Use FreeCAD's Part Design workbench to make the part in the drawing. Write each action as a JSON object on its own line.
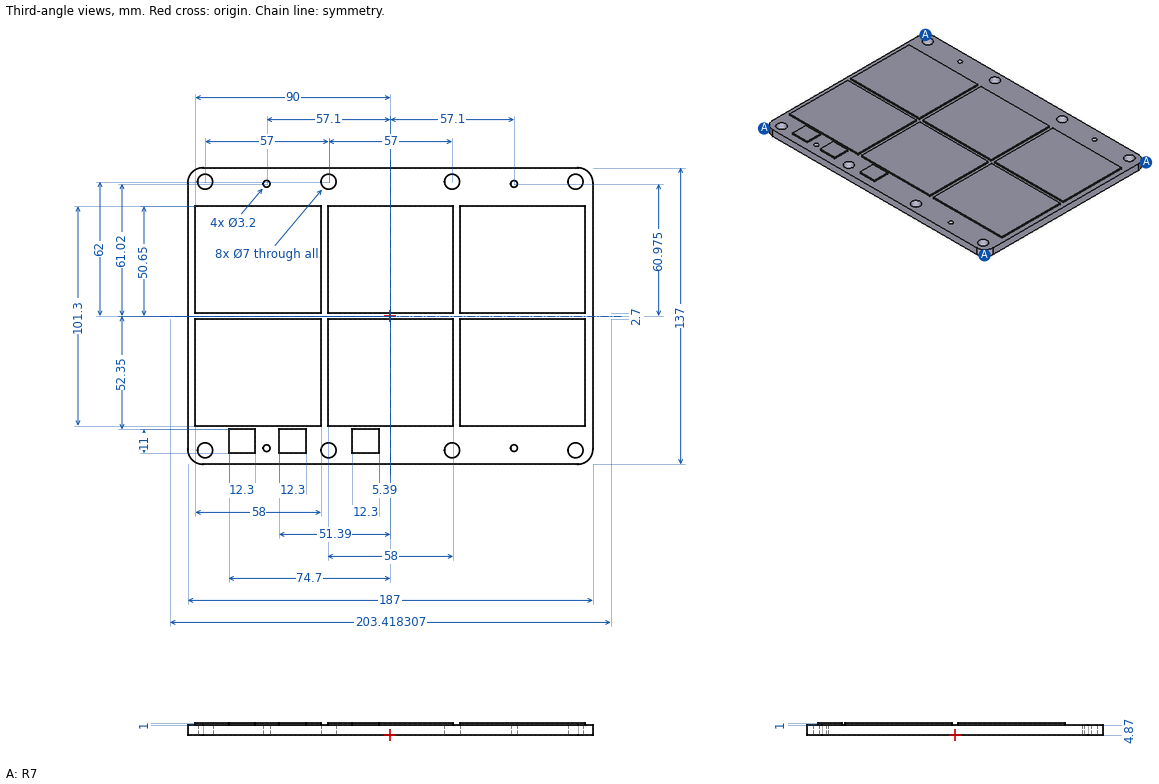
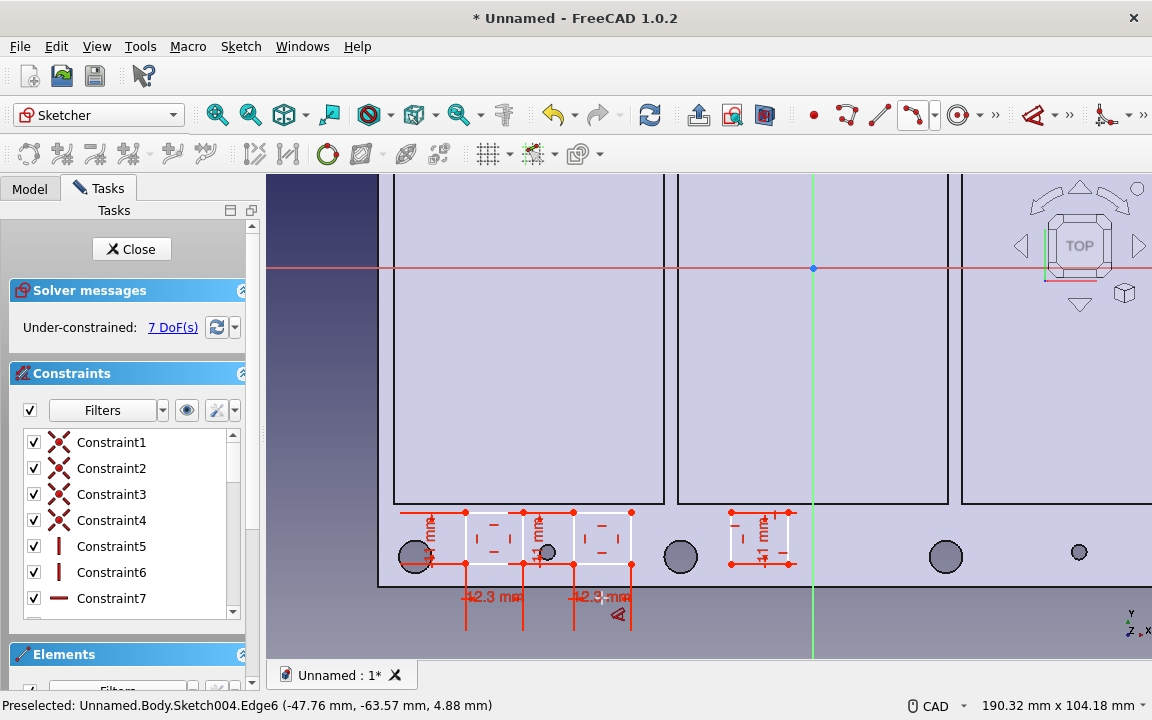
{"action": "left_click", "coordinate": [748, 564]}
{"action": "left_click", "coordinate": [760, 598]}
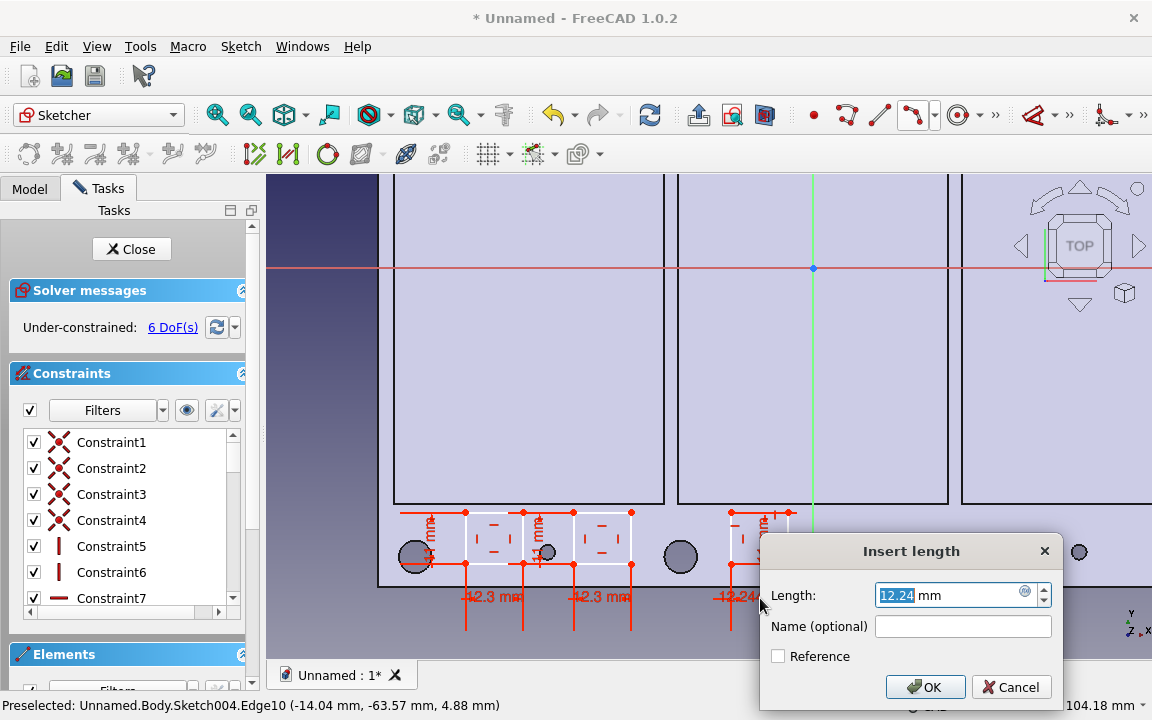
{"action": "type", "text": "12.3"}
{"action": "key", "text": "Return"}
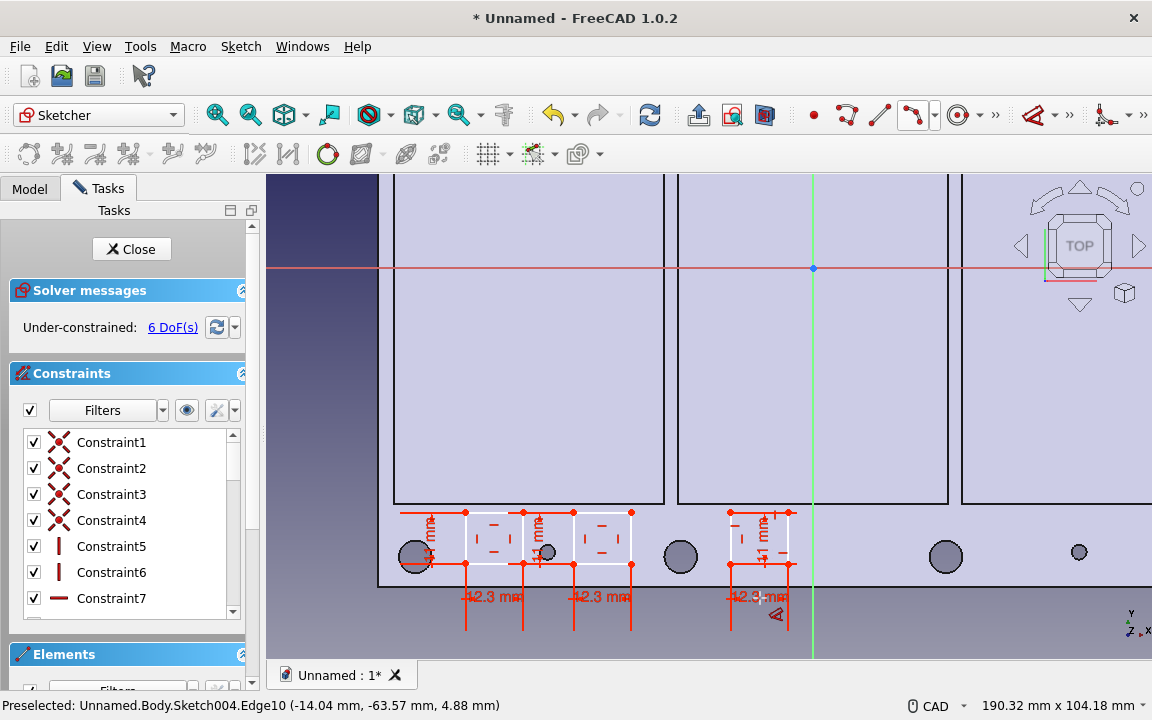
{"action": "left_click", "coordinate": [466, 513]}
{"action": "left_click", "coordinate": [640, 234]}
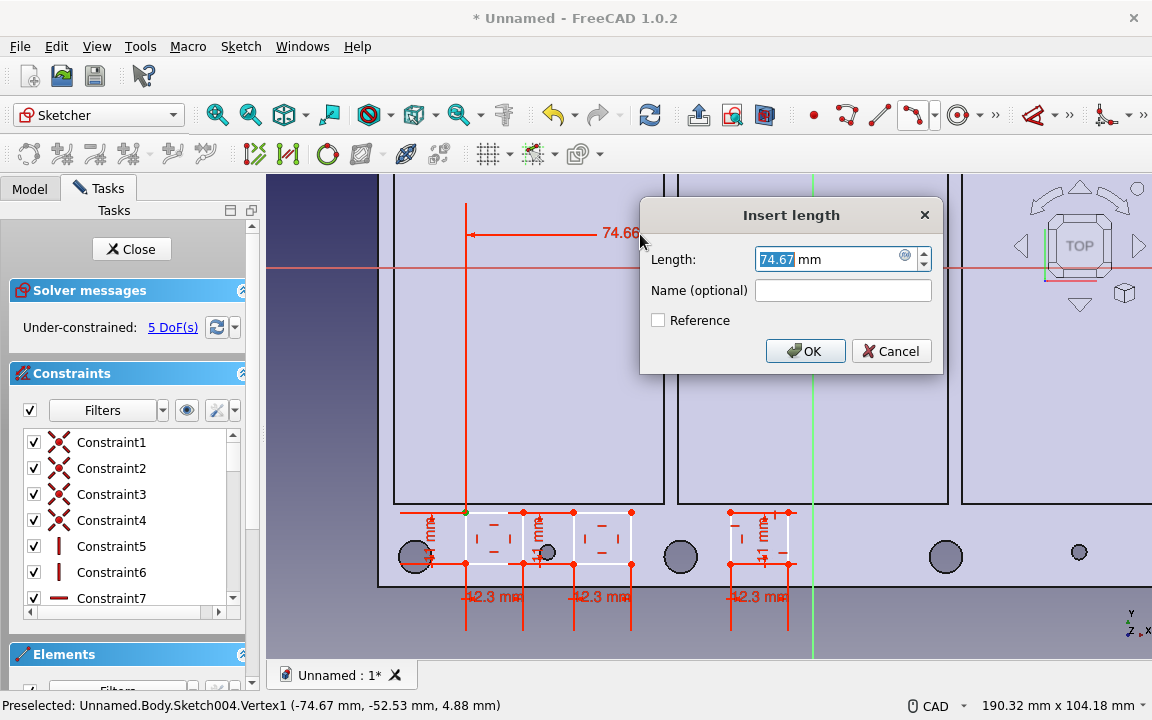
{"action": "type", "text": "74.7"}
{"action": "key", "text": "Return"}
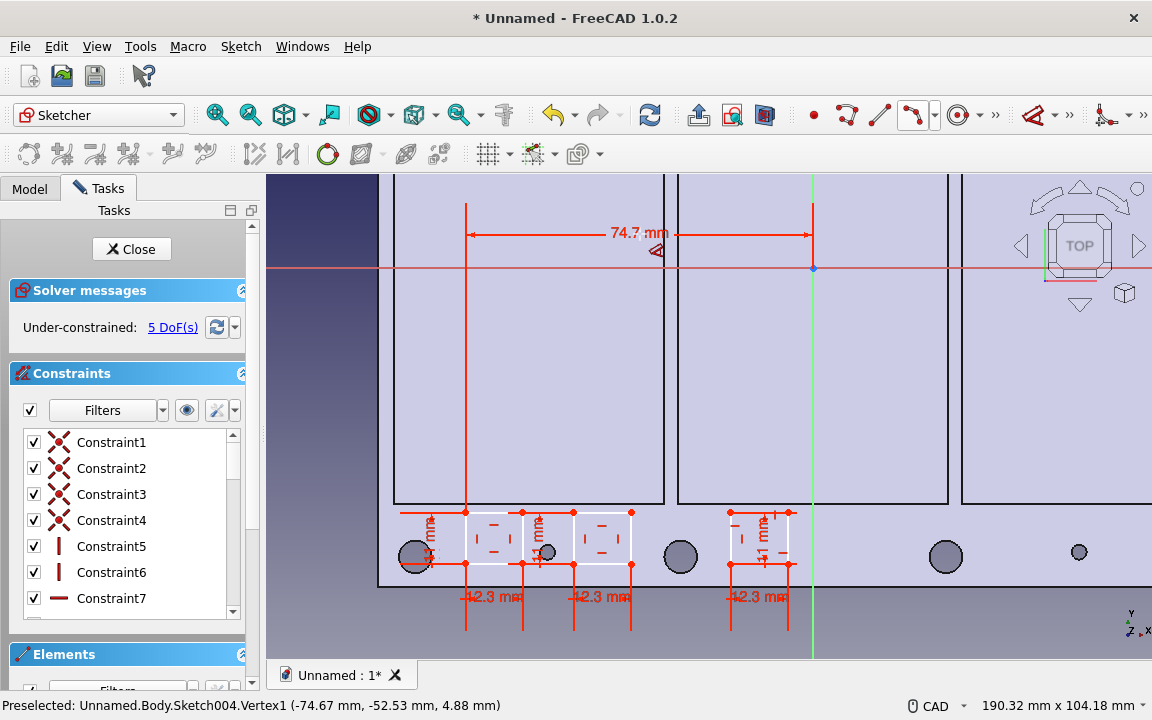
{"action": "scroll", "coordinate": [788, 564], "scroll_direction": "up", "scroll_amount": 3}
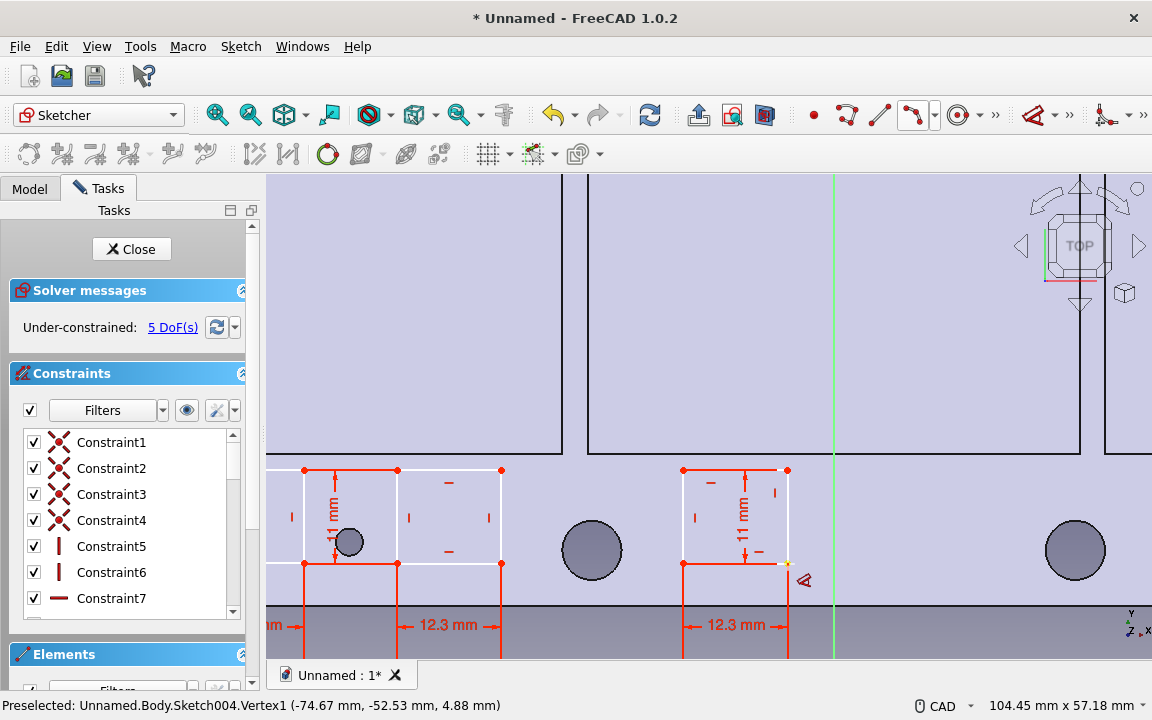
{"action": "left_click", "coordinate": [788, 564]}
{"action": "left_click", "coordinate": [811, 598]}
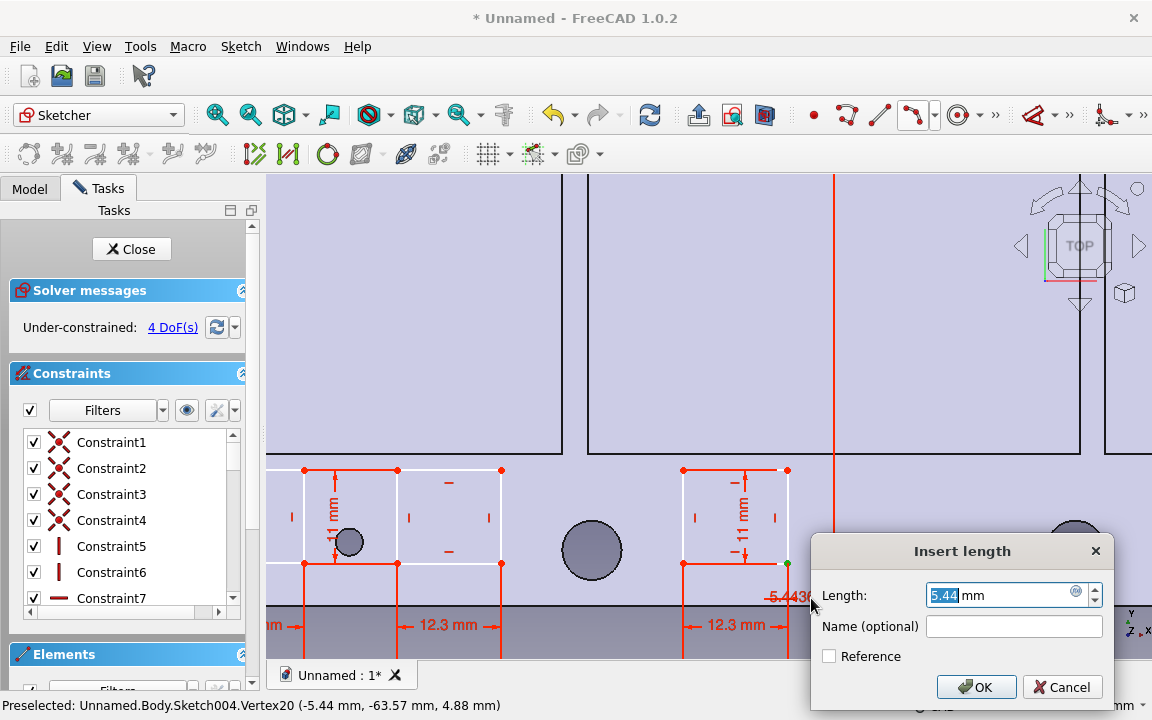
{"action": "type", "text": "5.39"}
{"action": "key", "text": "Return"}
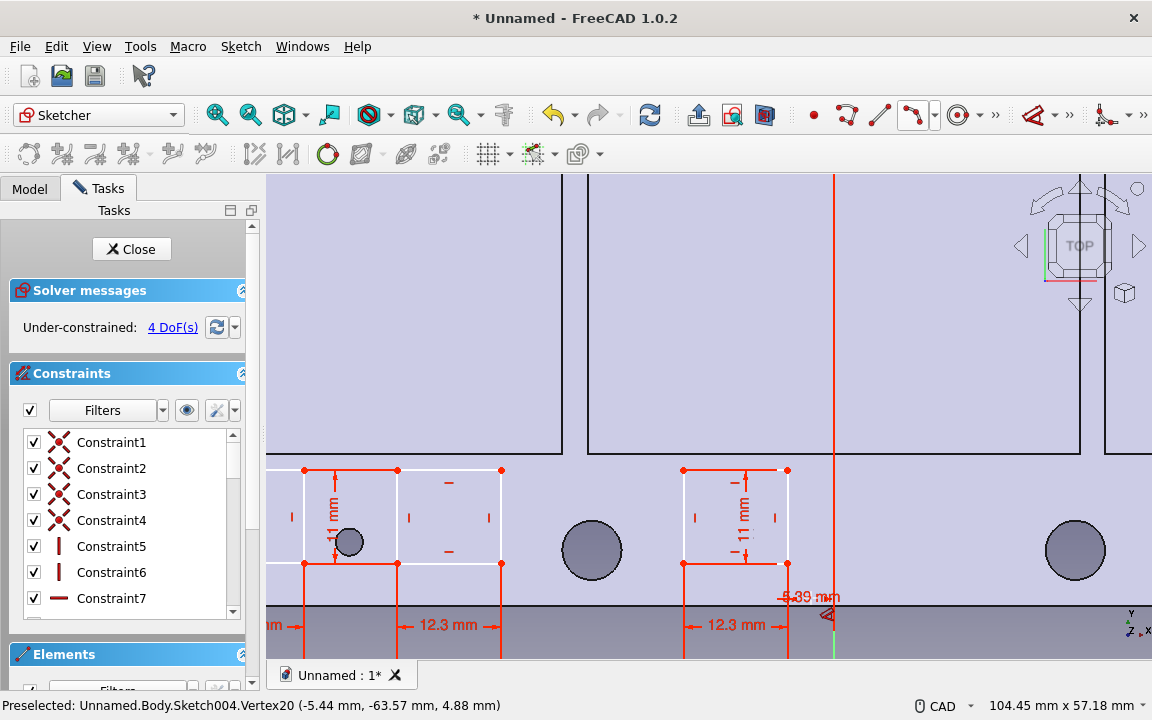
{"action": "scroll", "coordinate": [791, 567], "scroll_direction": "down", "scroll_amount": 3}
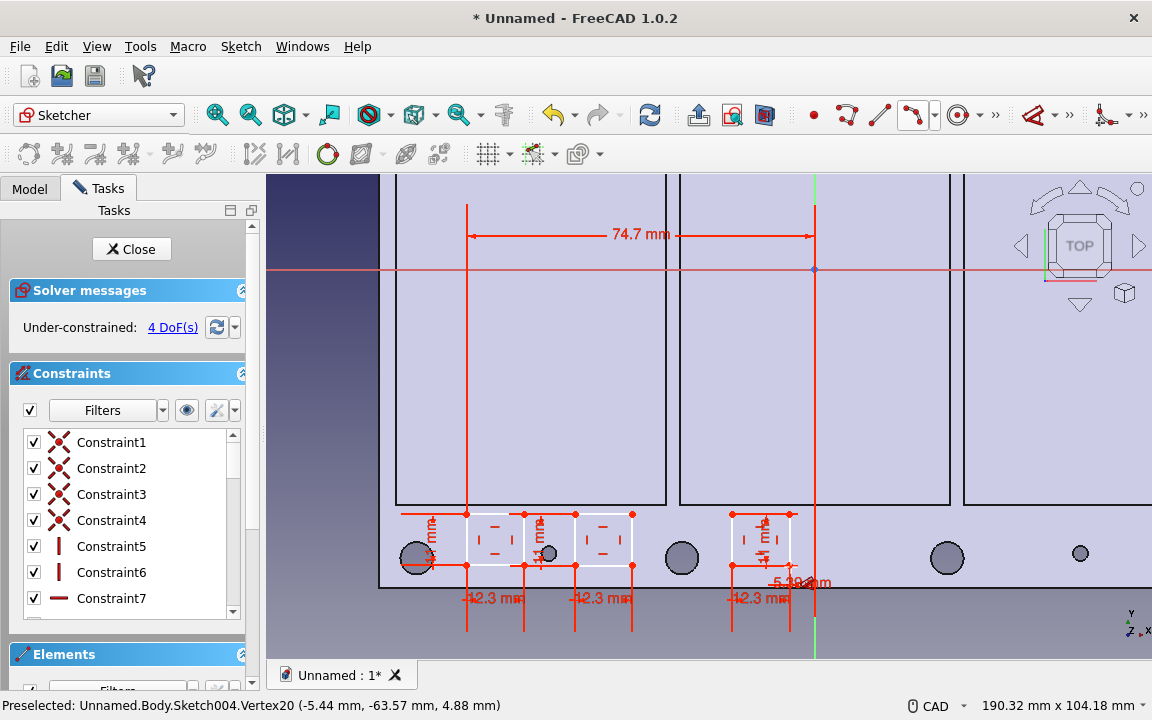
{"action": "left_click", "coordinate": [467, 514]}
{"action": "left_click", "coordinate": [849, 392]}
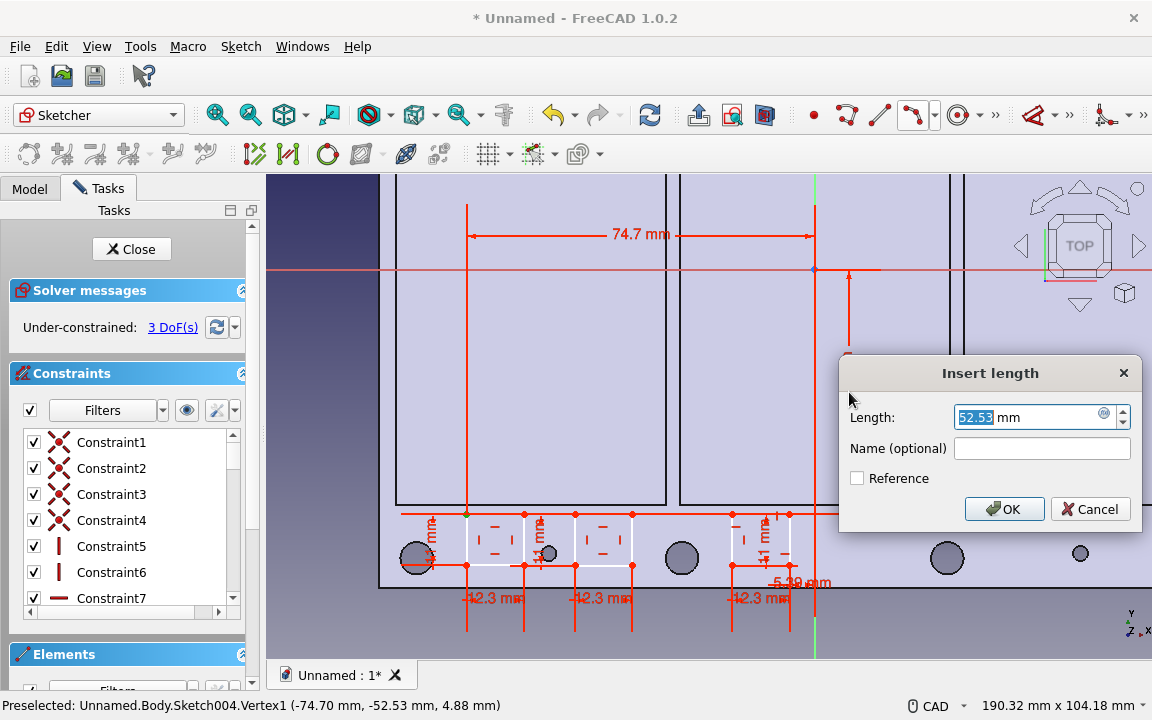
{"action": "type", "text": "52.35"}
{"action": "key", "text": "Return"}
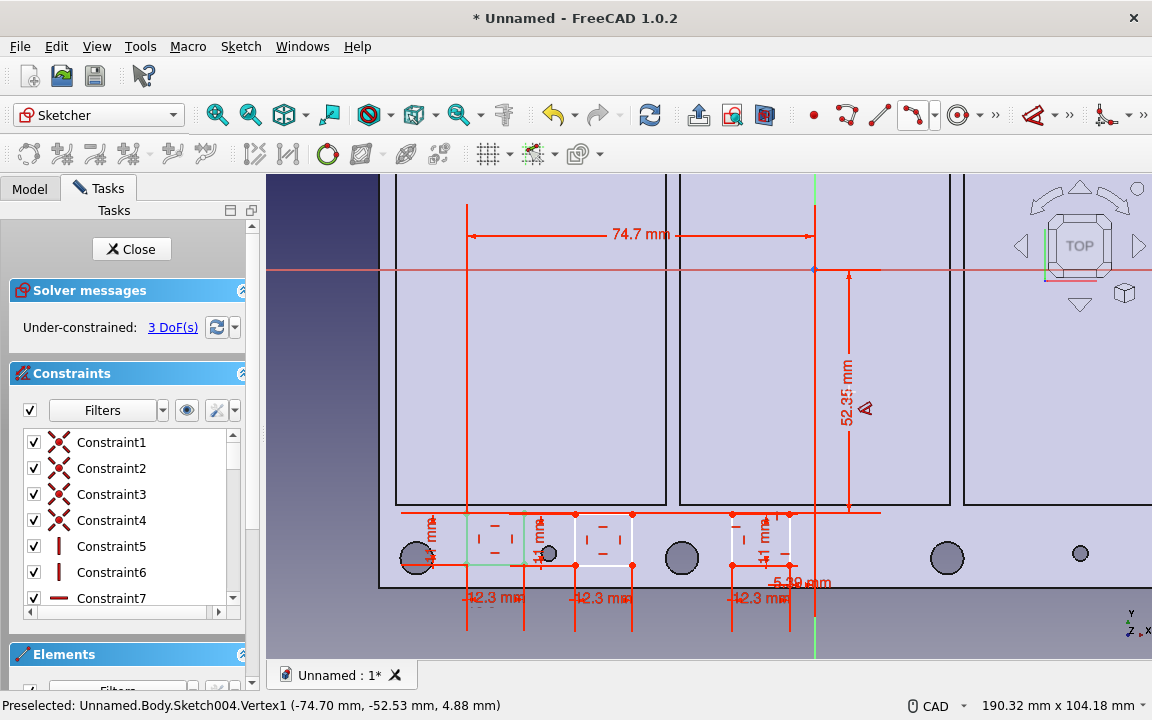
{"action": "left_click", "coordinate": [575, 514]}
{"action": "left_click", "coordinate": [750, 236]}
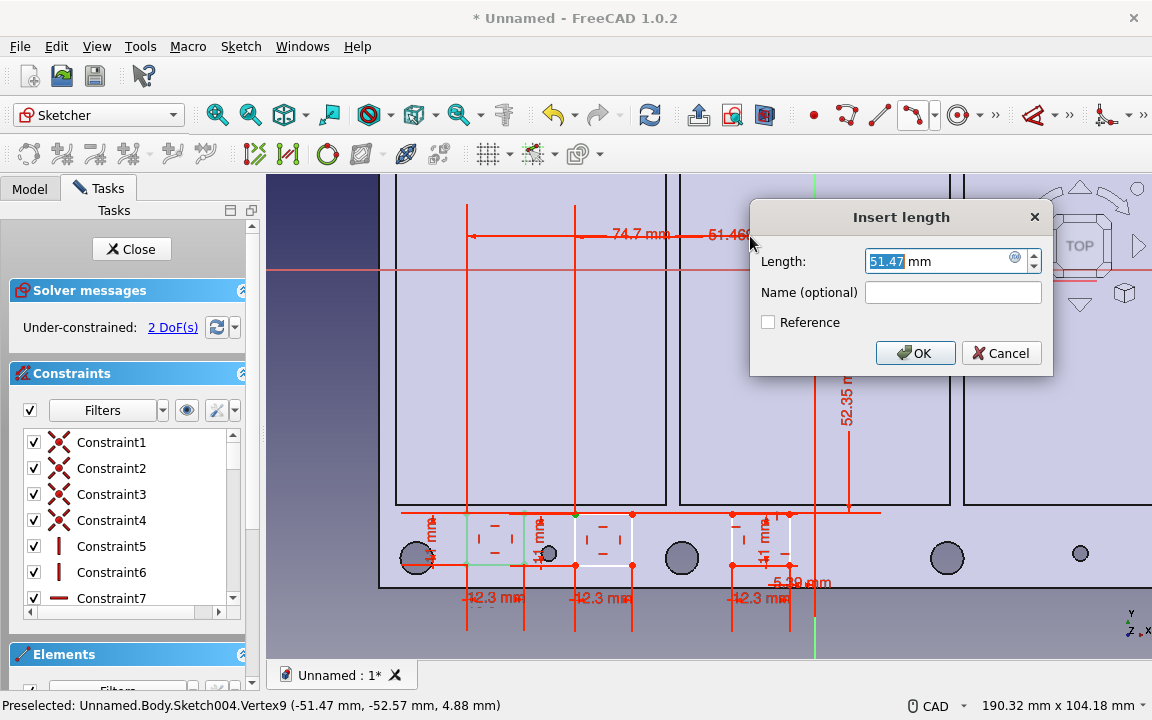
{"action": "type", "text": "51.39"}
{"action": "key", "text": "Return"}